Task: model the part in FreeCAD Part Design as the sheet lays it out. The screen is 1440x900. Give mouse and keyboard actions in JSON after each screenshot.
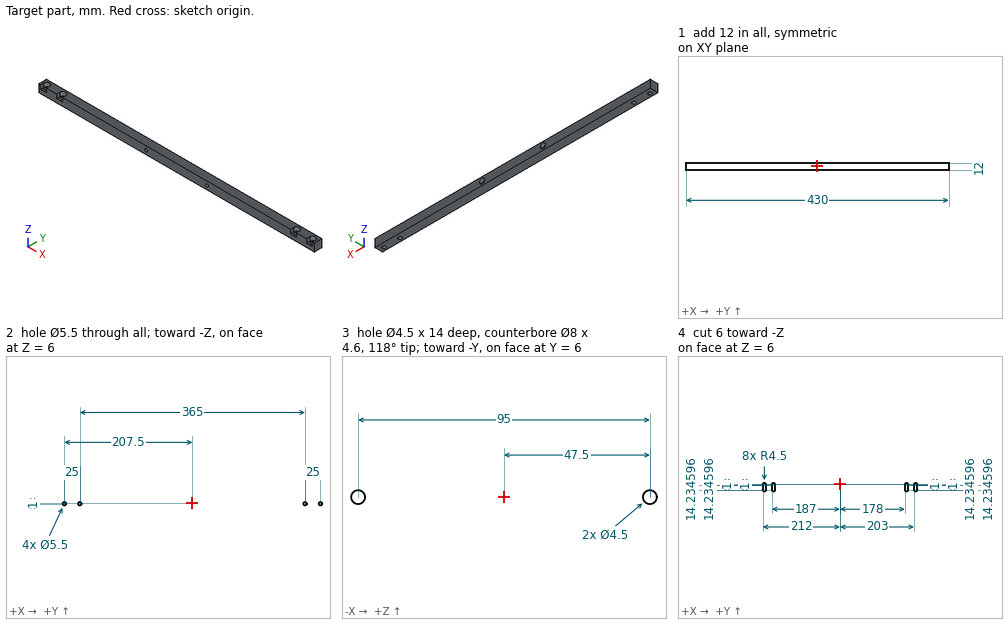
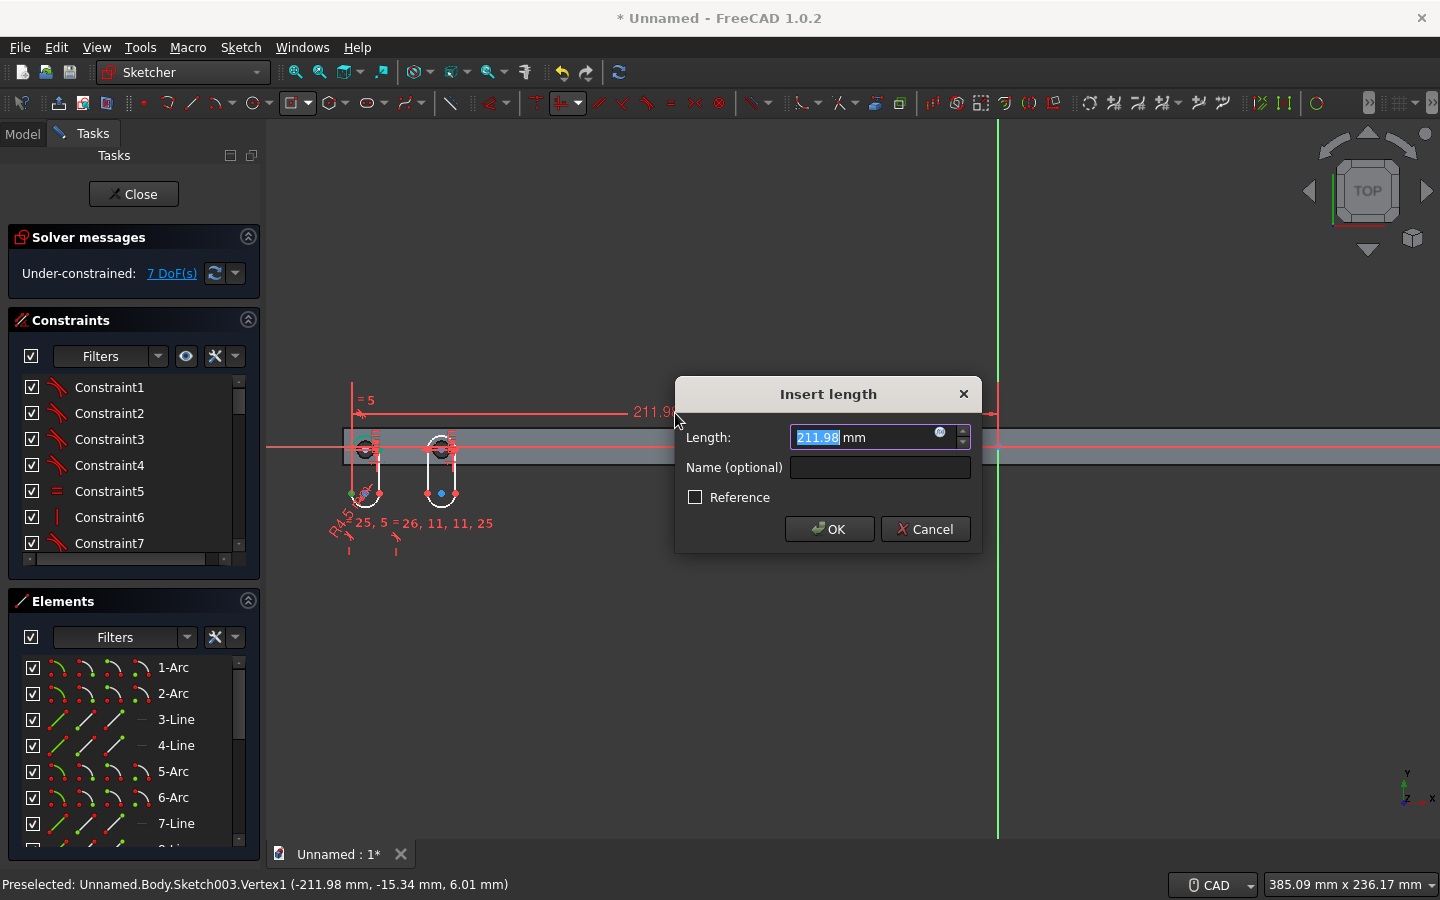
{"action": "type", "text": "212"}
{"action": "key", "text": "Return"}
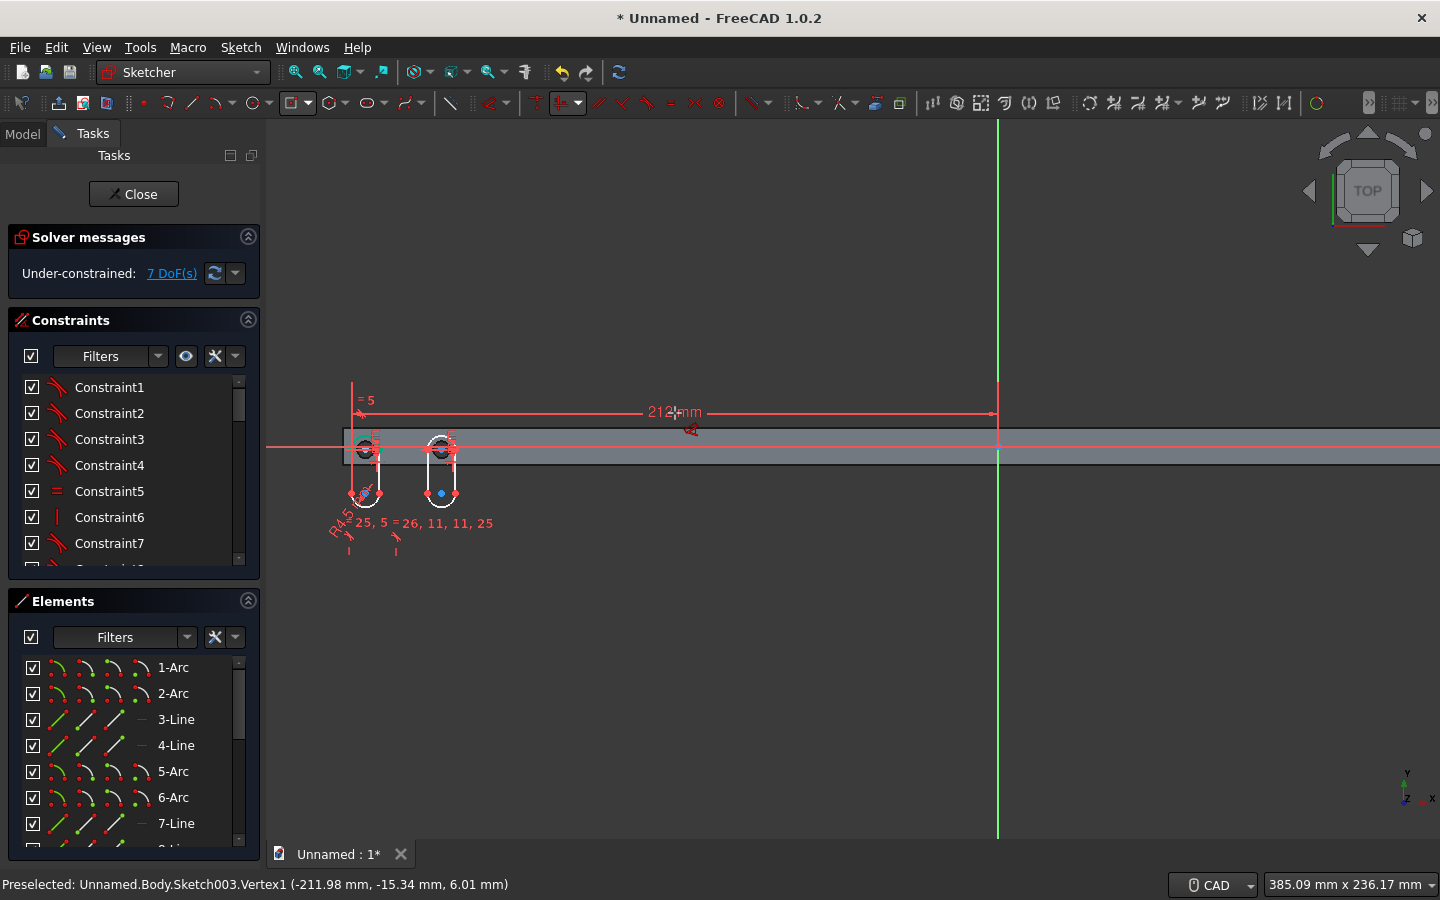
{"action": "left_click", "coordinate": [428, 494]}
{"action": "left_click", "coordinate": [582, 413]}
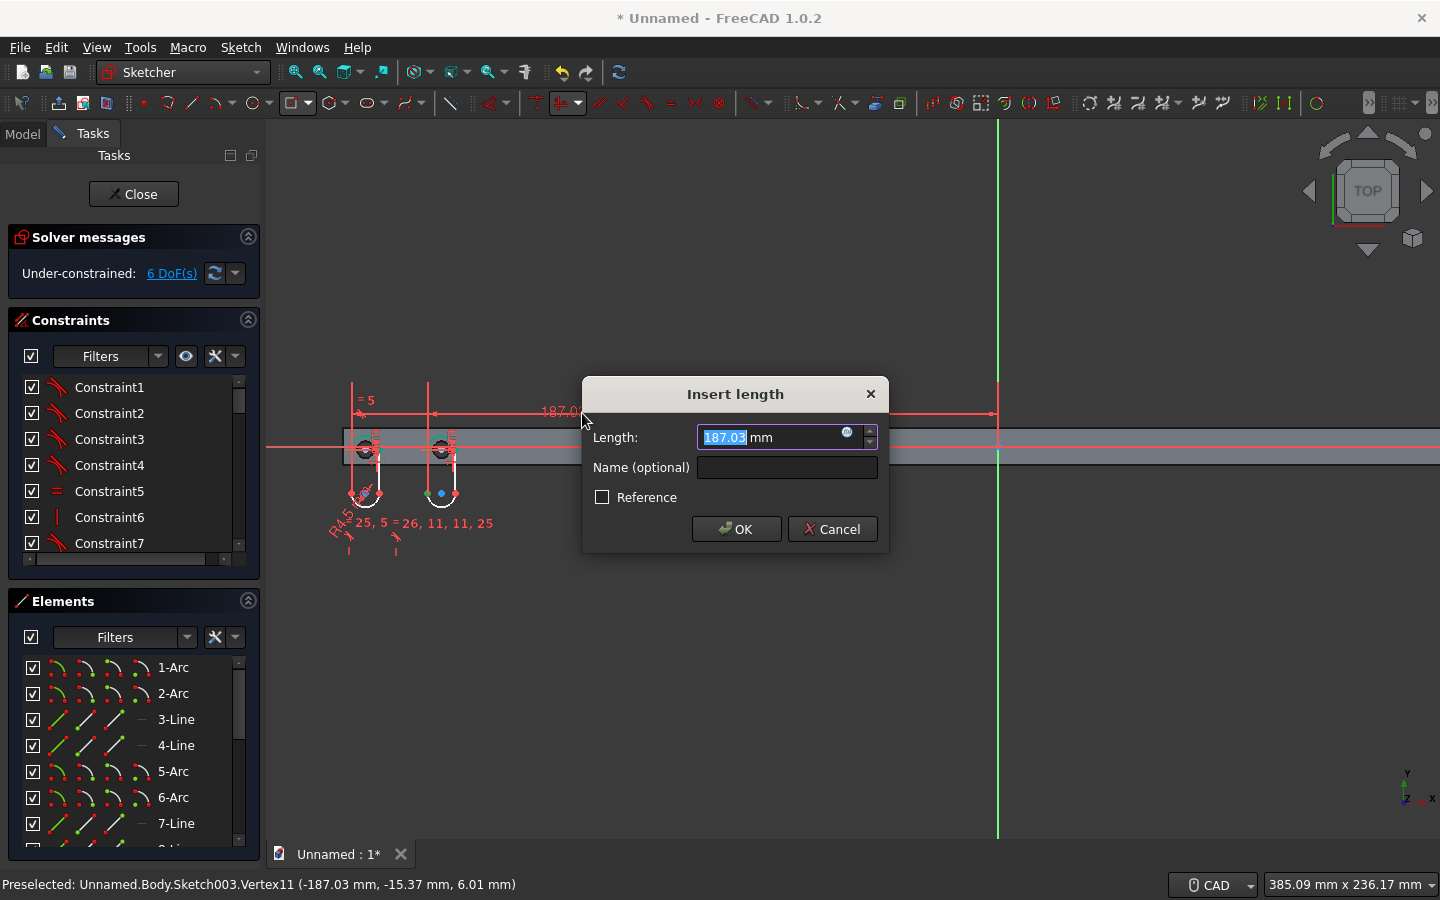
{"action": "type", "text": "187"}
{"action": "key", "text": "Return"}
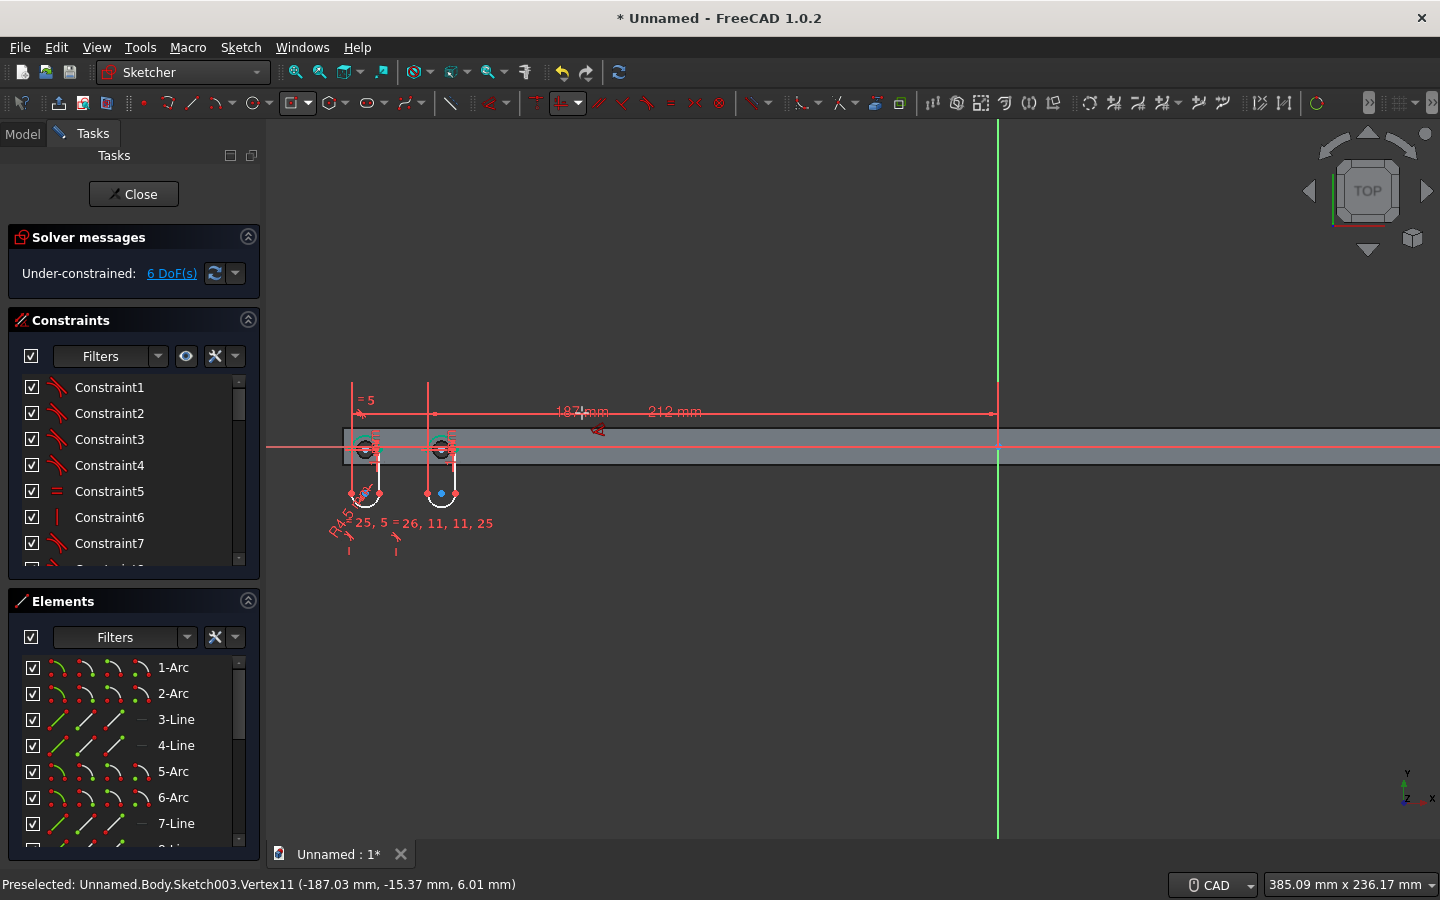
{"action": "scroll", "coordinate": [525, 488], "scroll_direction": "down", "scroll_amount": 3}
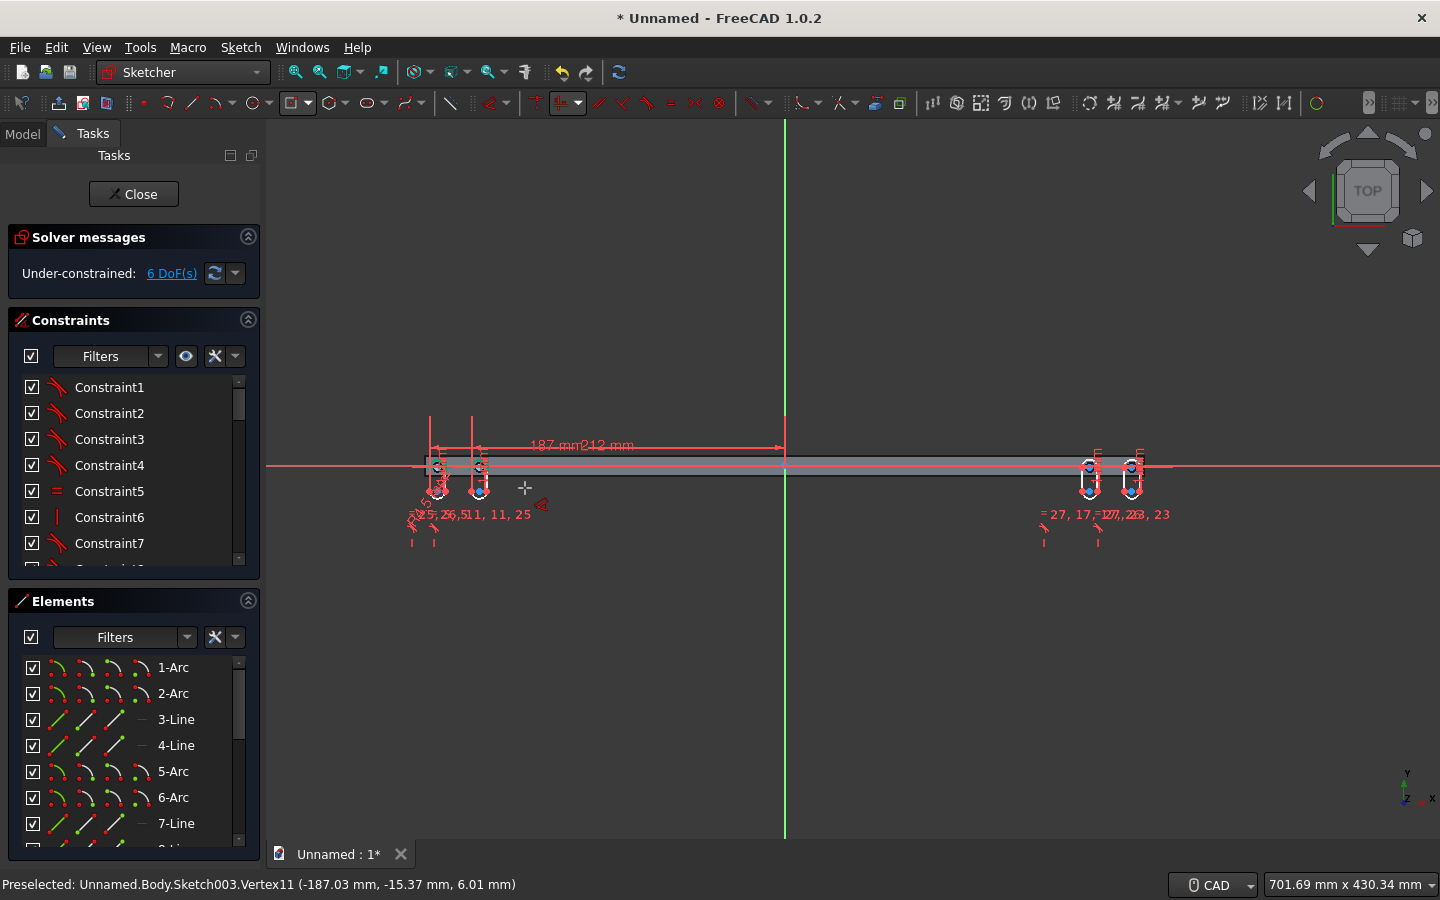
{"action": "scroll", "coordinate": [1082, 491], "scroll_direction": "up", "scroll_amount": 3}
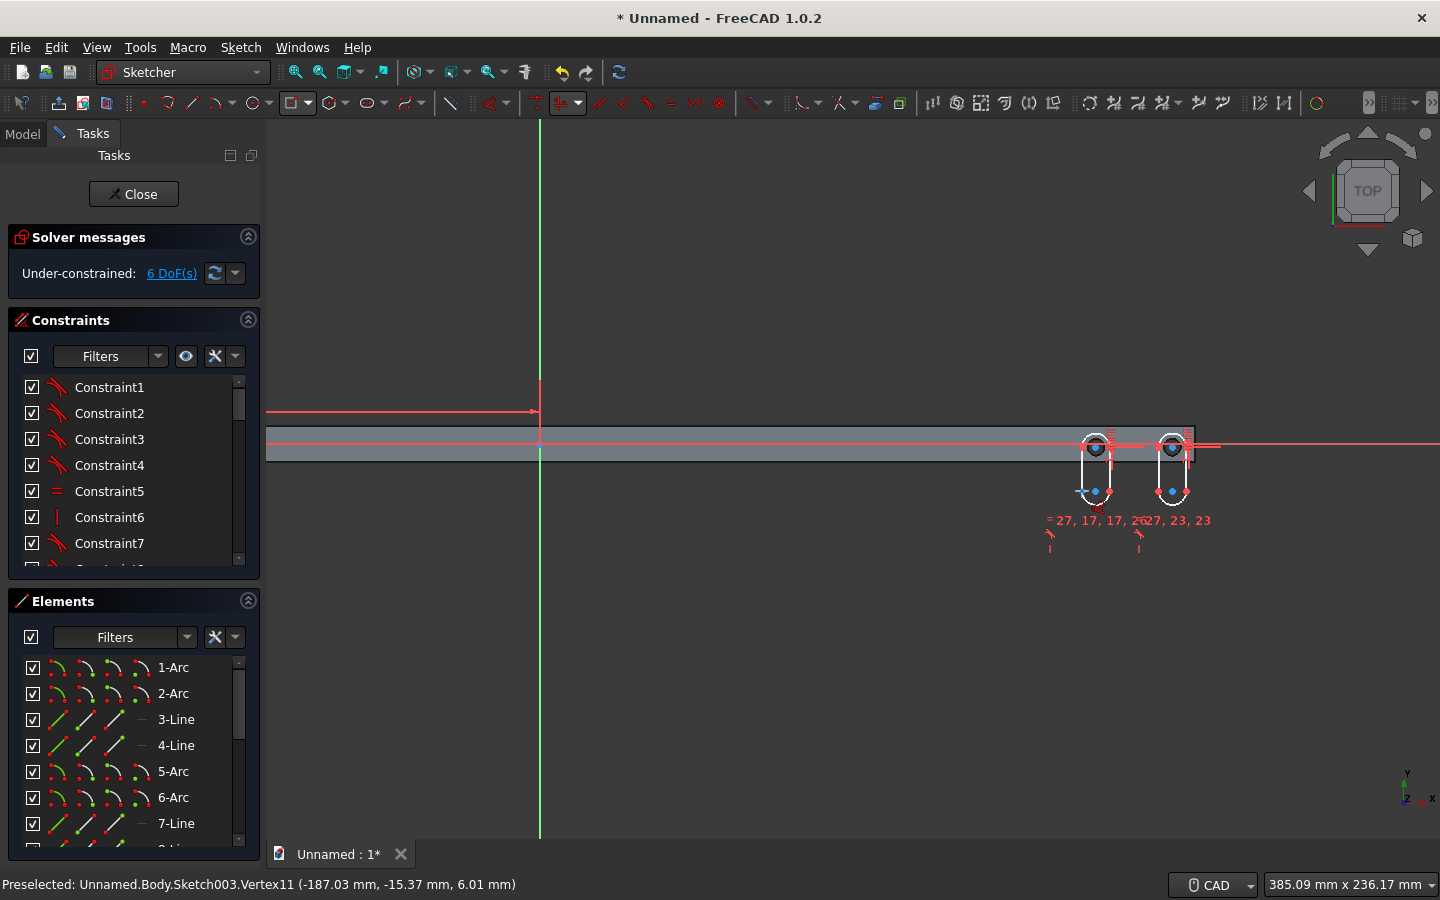
{"action": "left_click", "coordinate": [1082, 491]}
{"action": "left_click", "coordinate": [811, 410]}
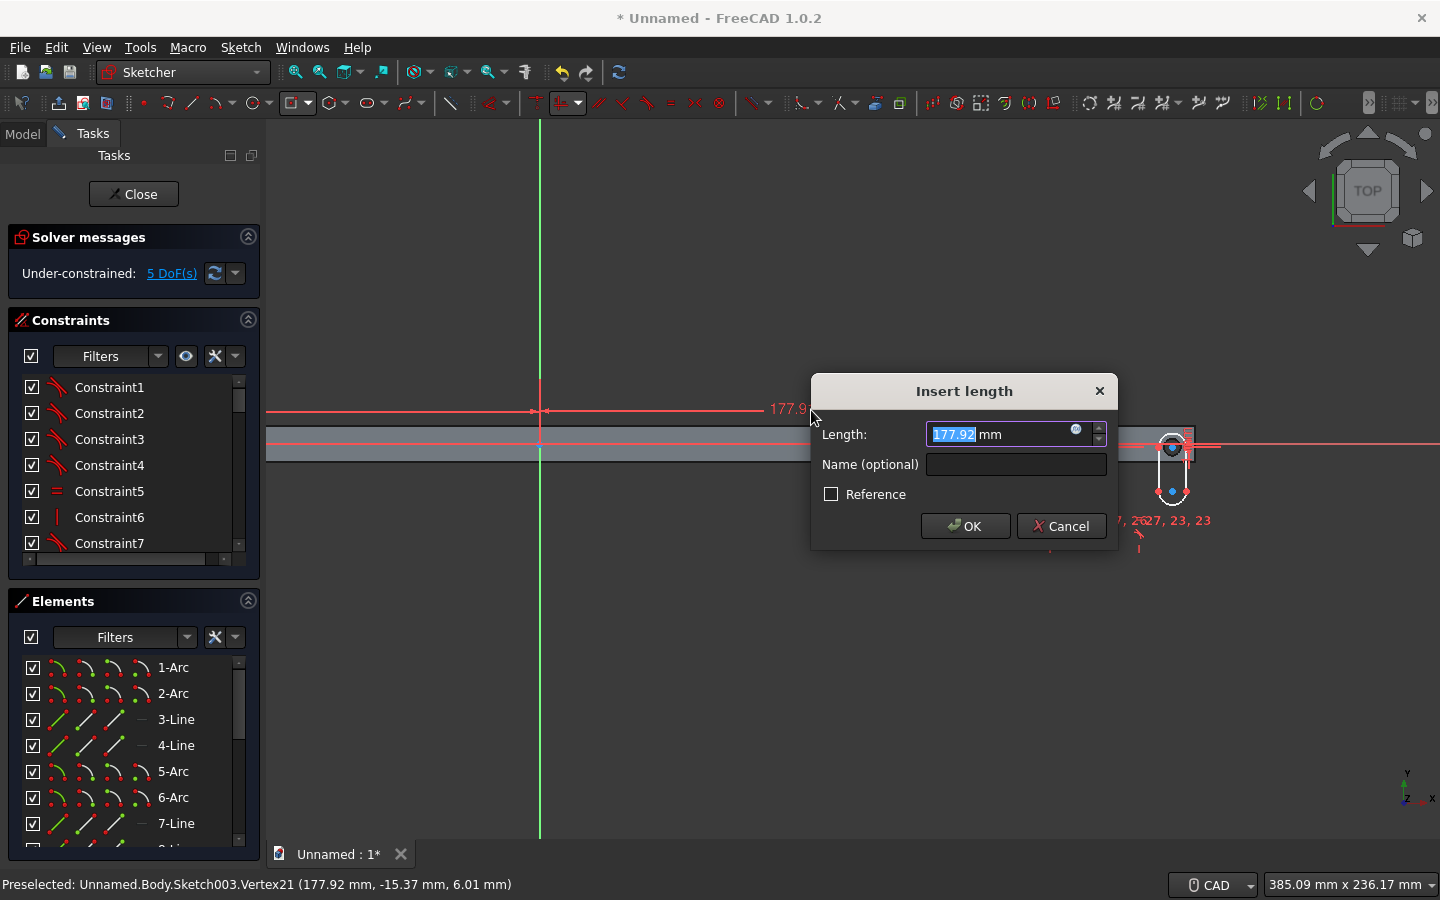
{"action": "type", "text": "178"}
{"action": "key", "text": "Return"}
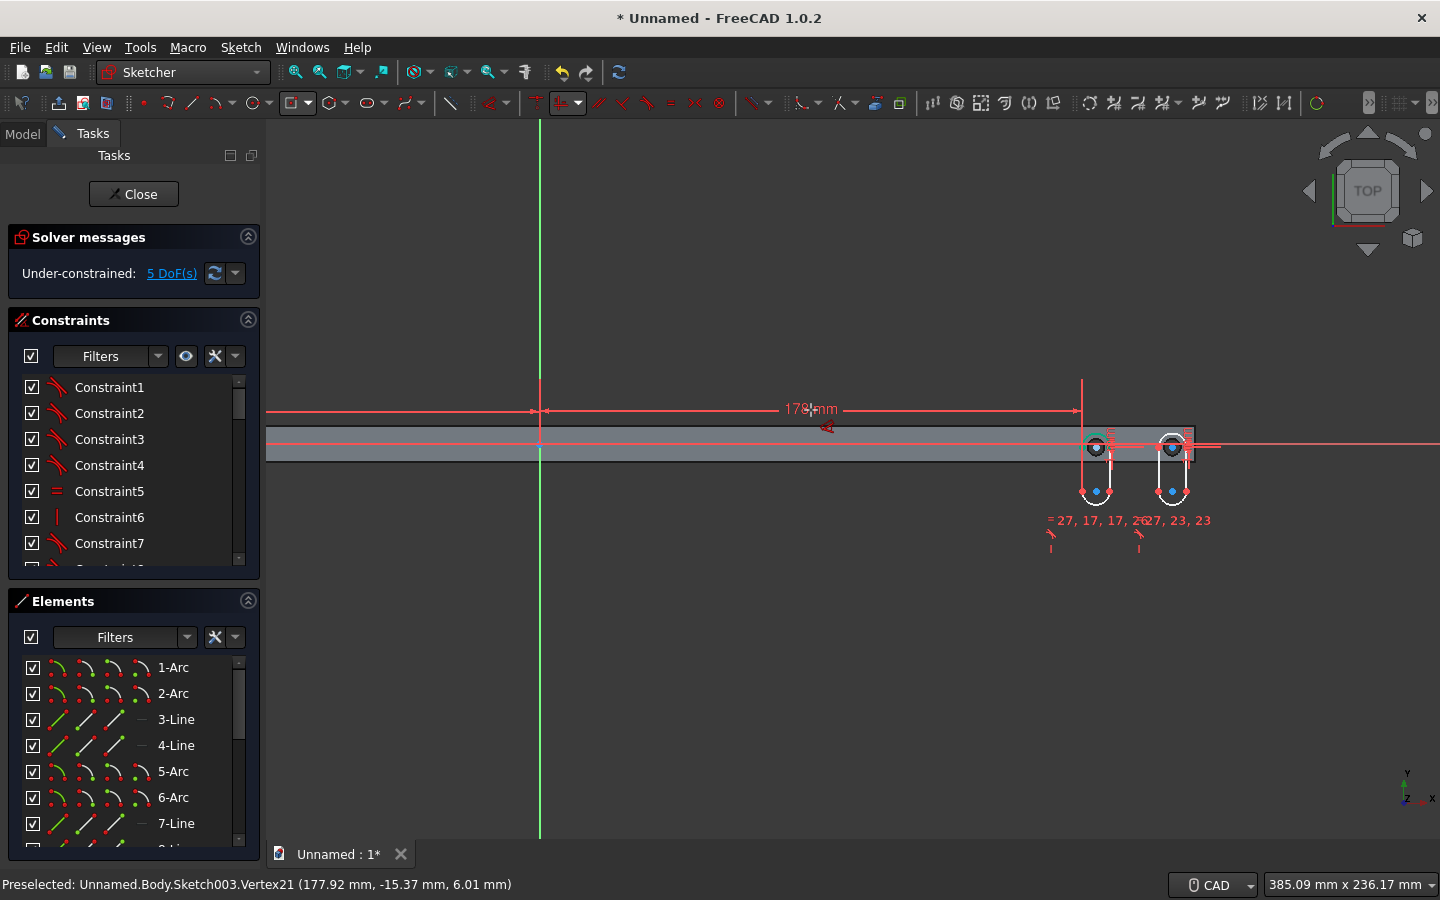
{"action": "left_click", "coordinate": [1159, 491]}
{"action": "left_click", "coordinate": [707, 410]}